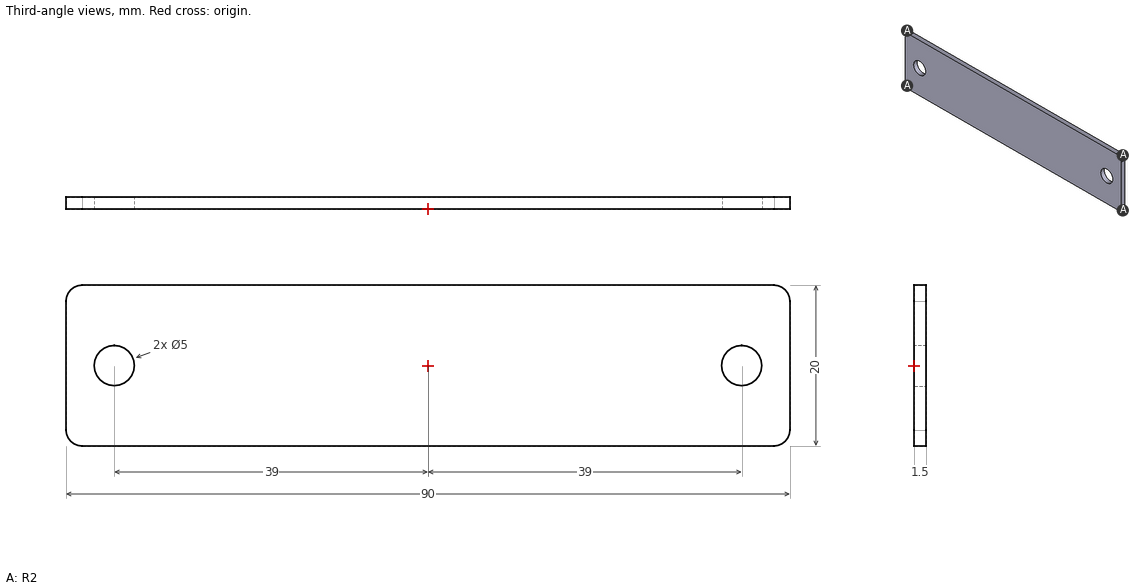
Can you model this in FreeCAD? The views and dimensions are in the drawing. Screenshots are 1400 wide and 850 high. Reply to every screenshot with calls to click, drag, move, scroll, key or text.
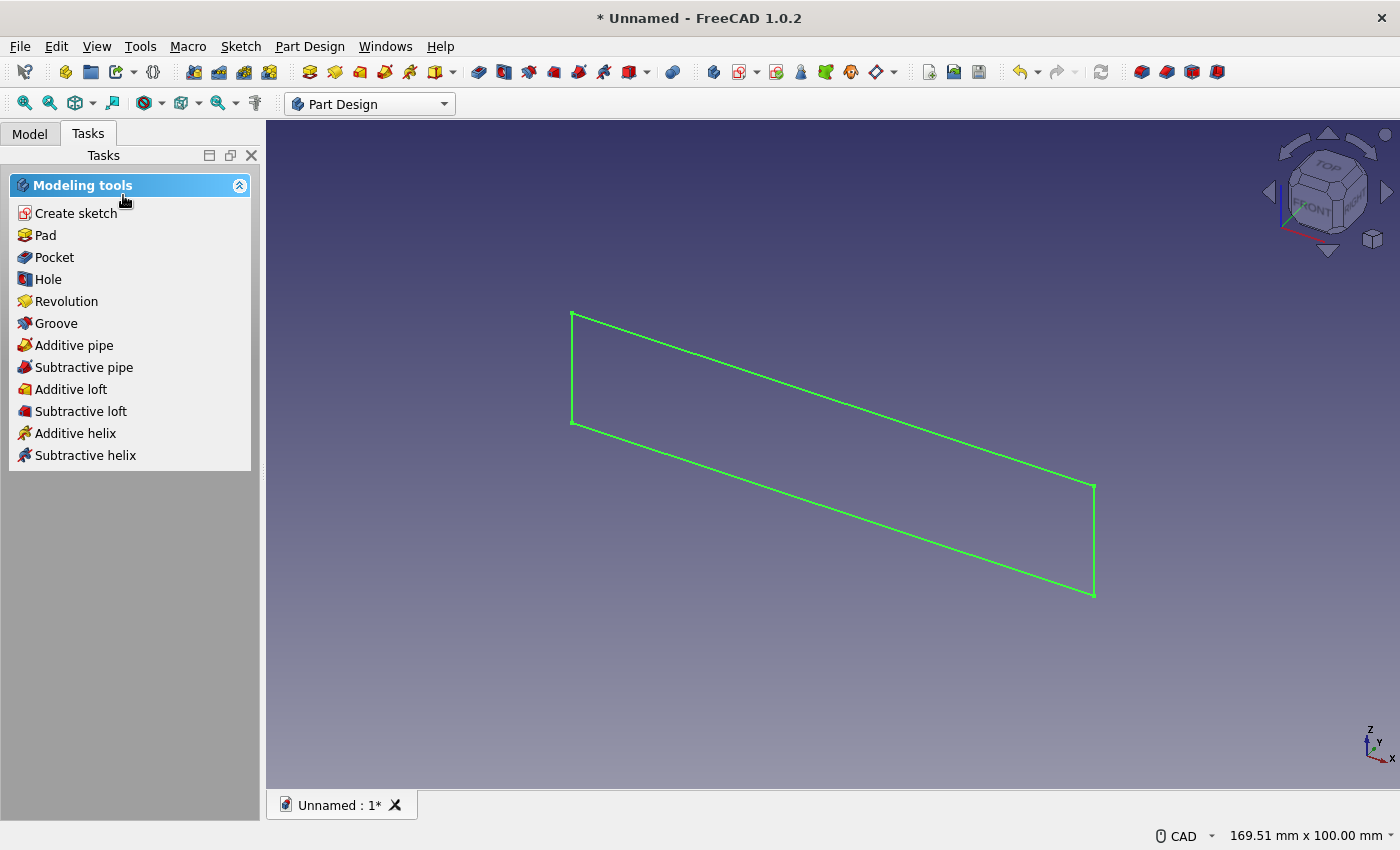
click(310, 72)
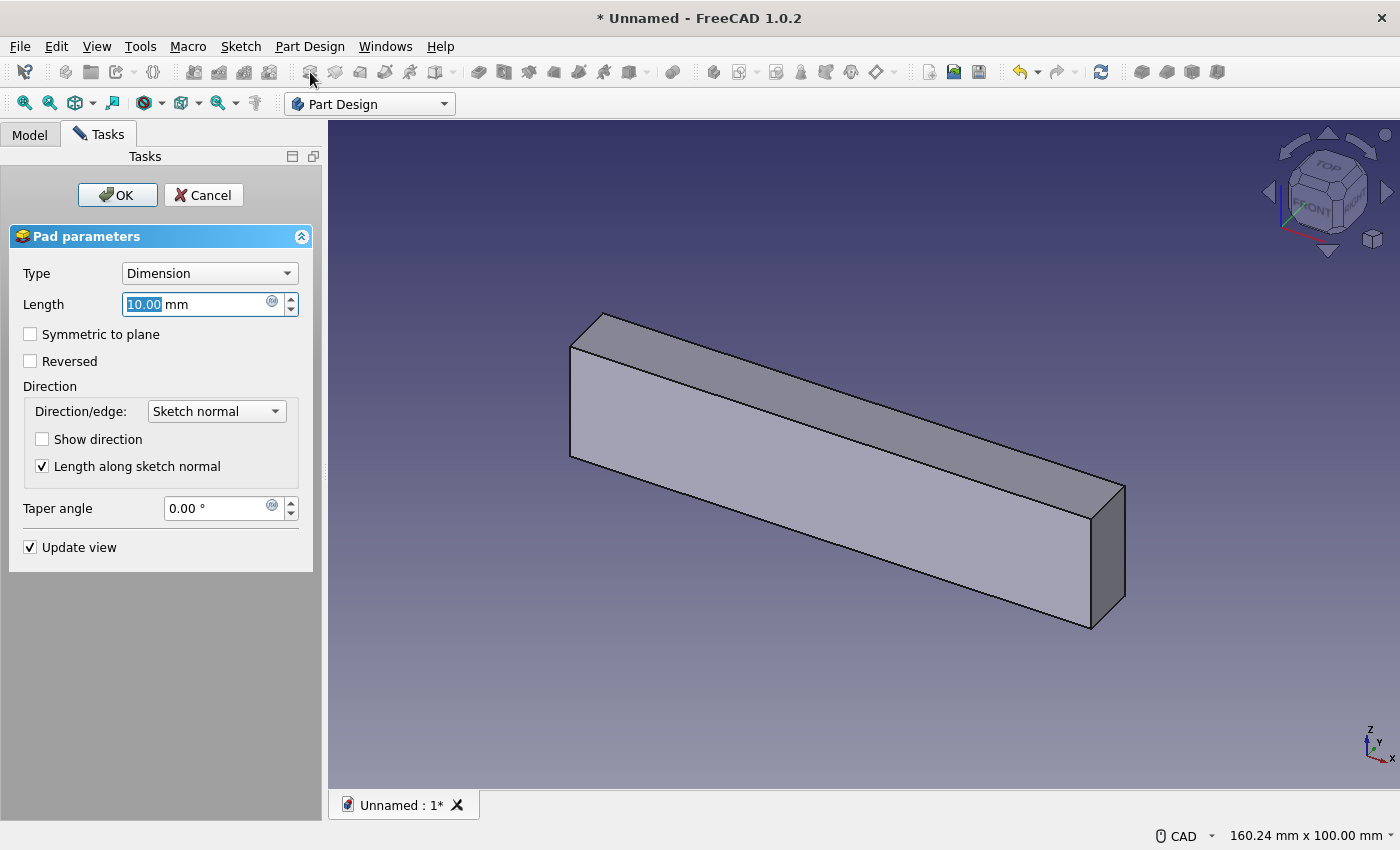
text(1.5)
key(Tab)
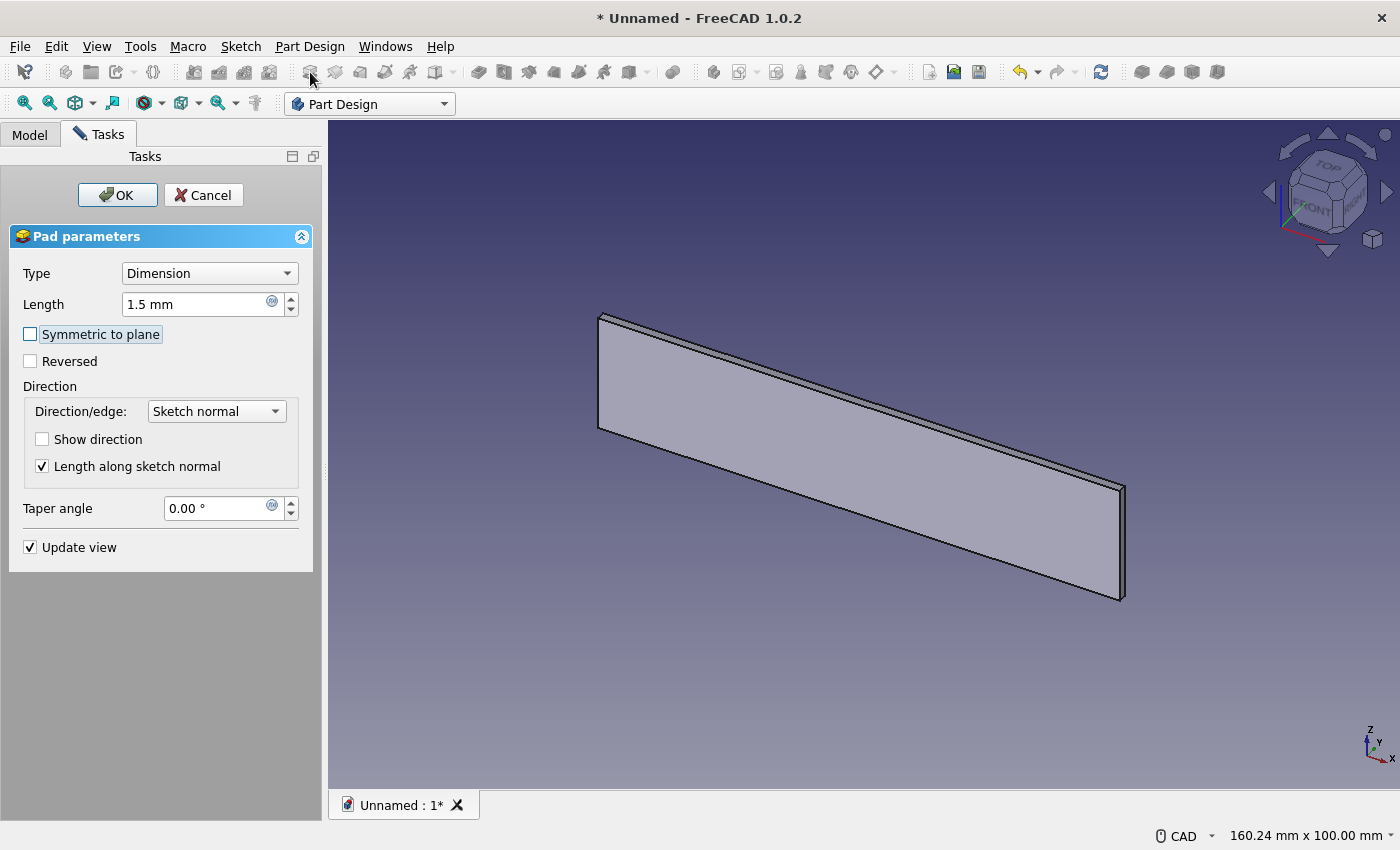
click(31, 361)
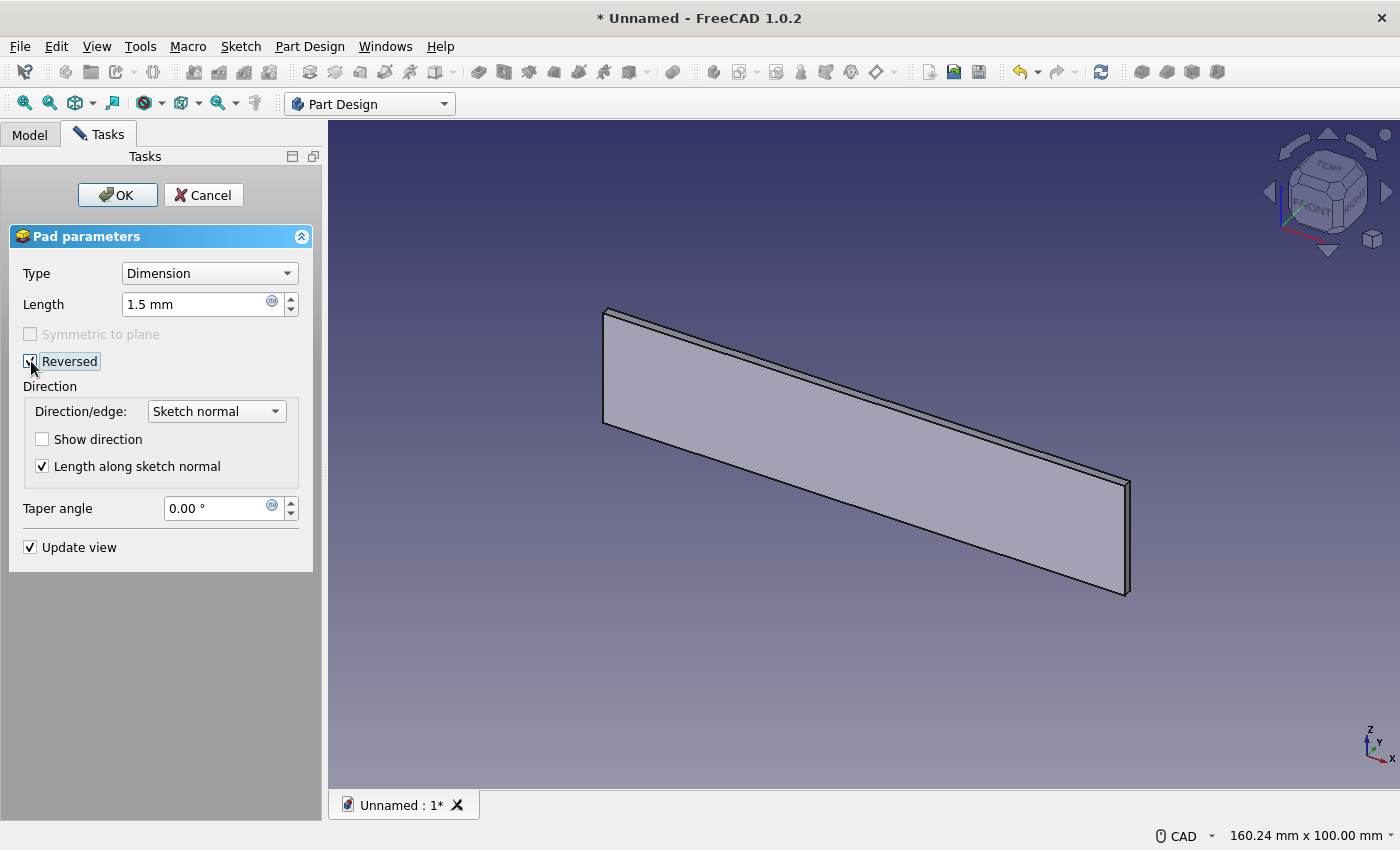
click(118, 195)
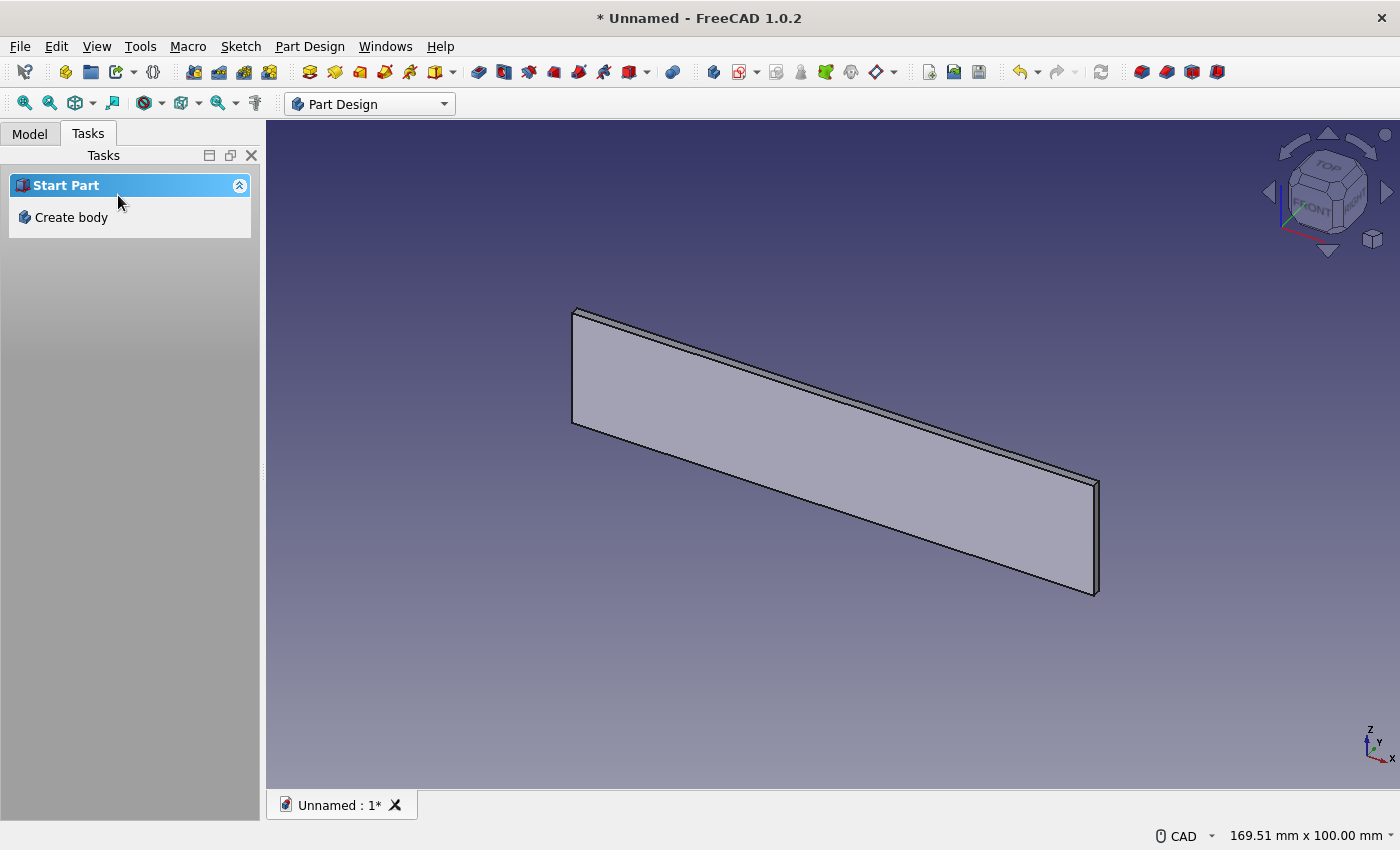
key(4)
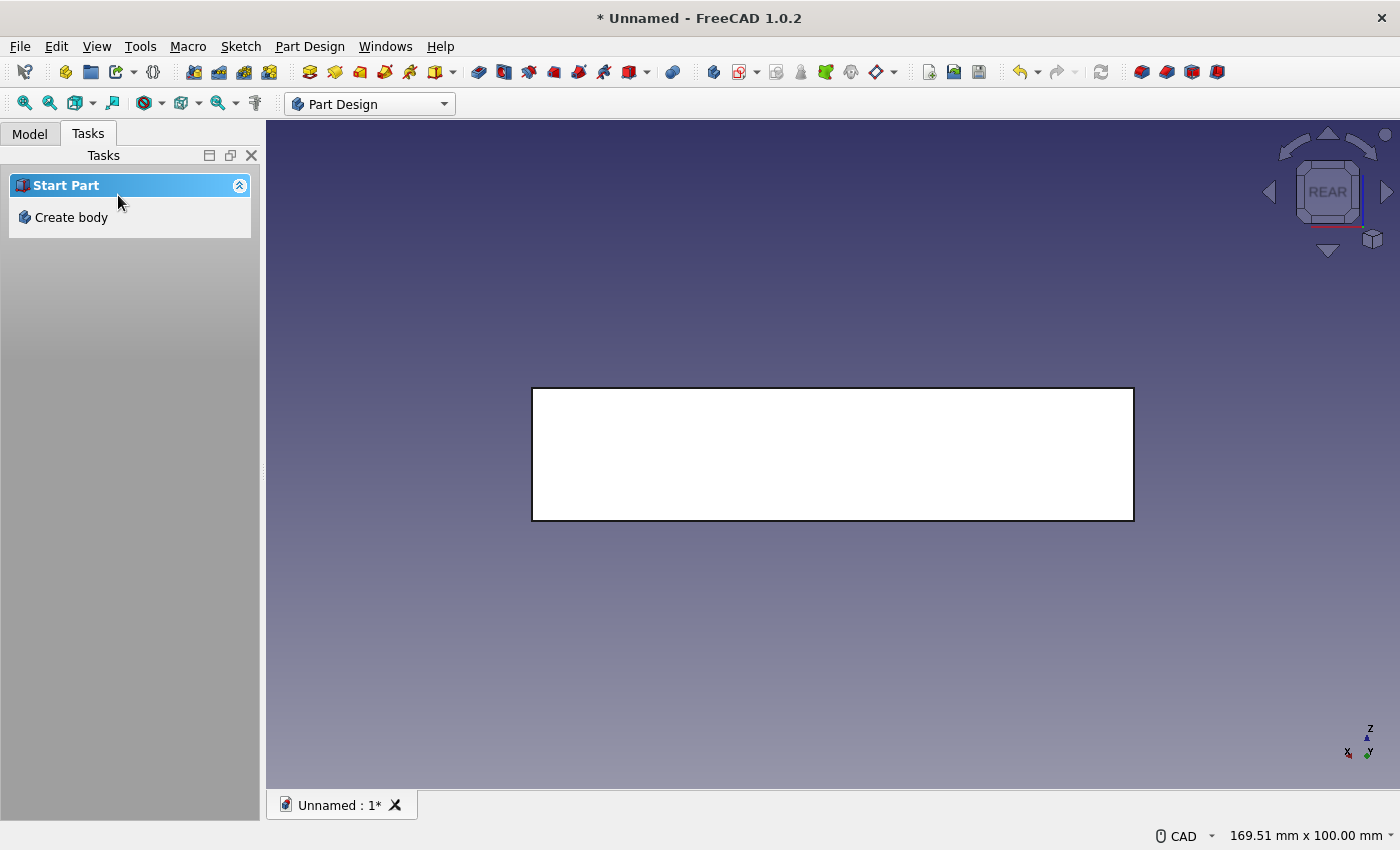
click(661, 453)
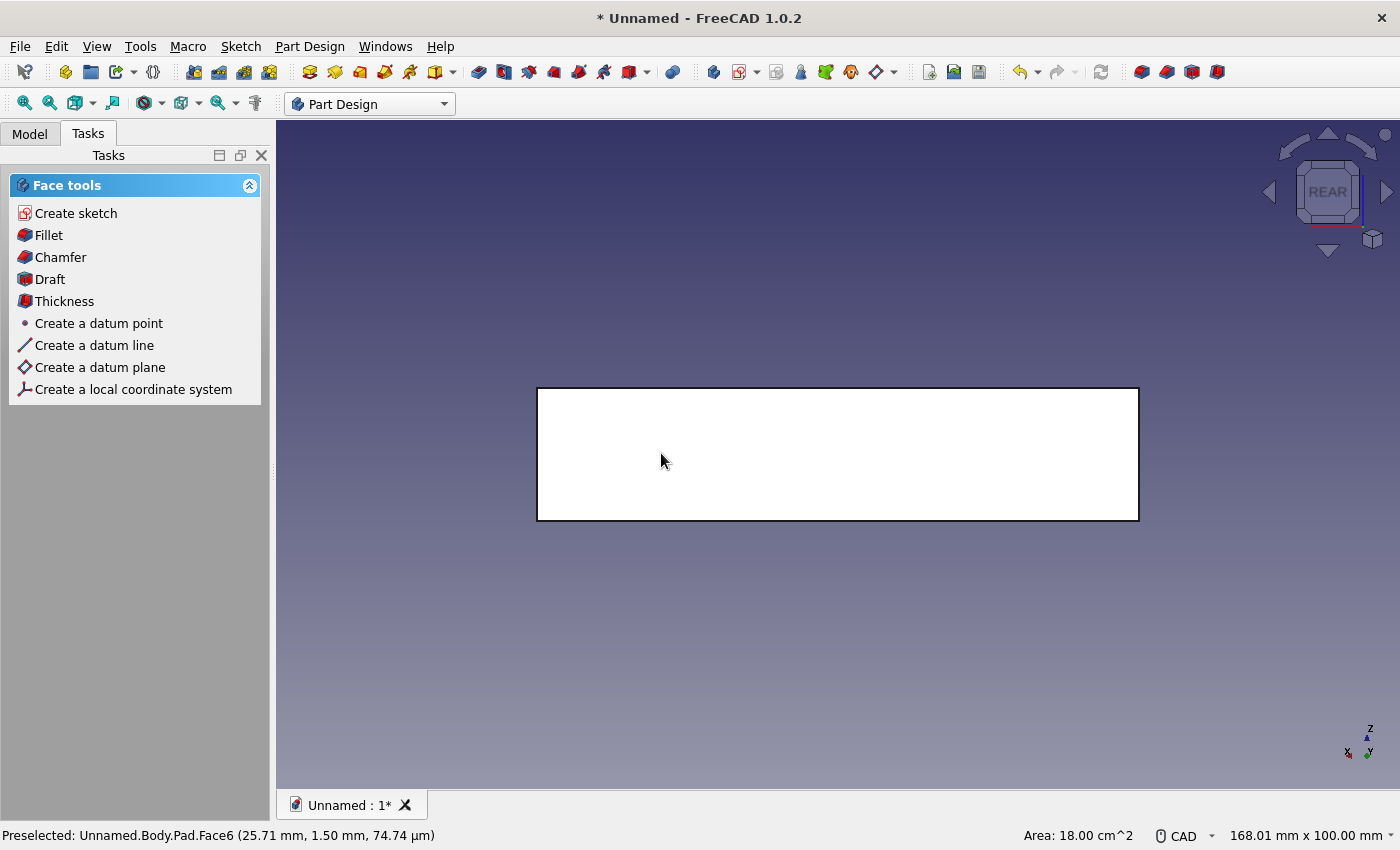
click(738, 72)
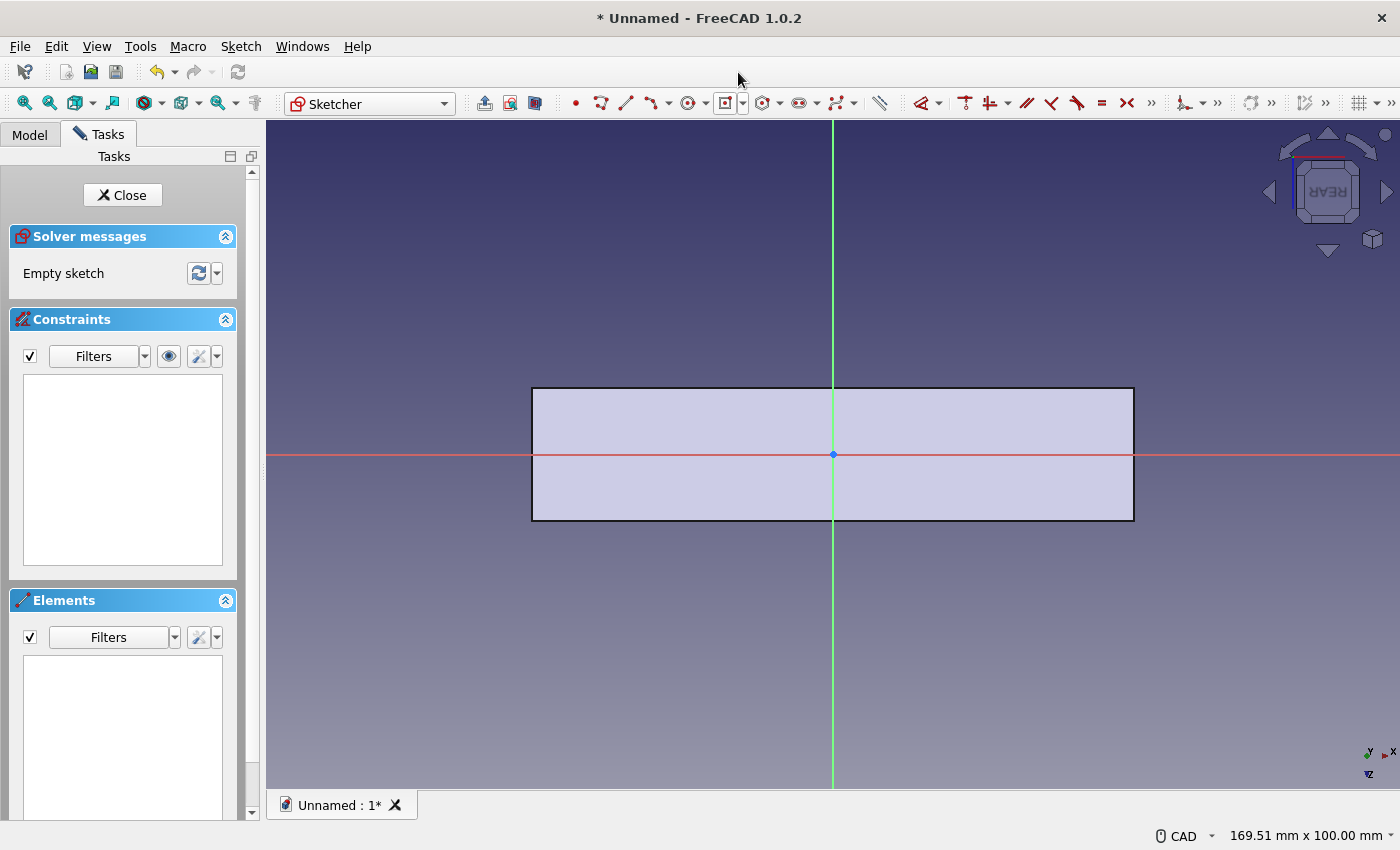
click(688, 104)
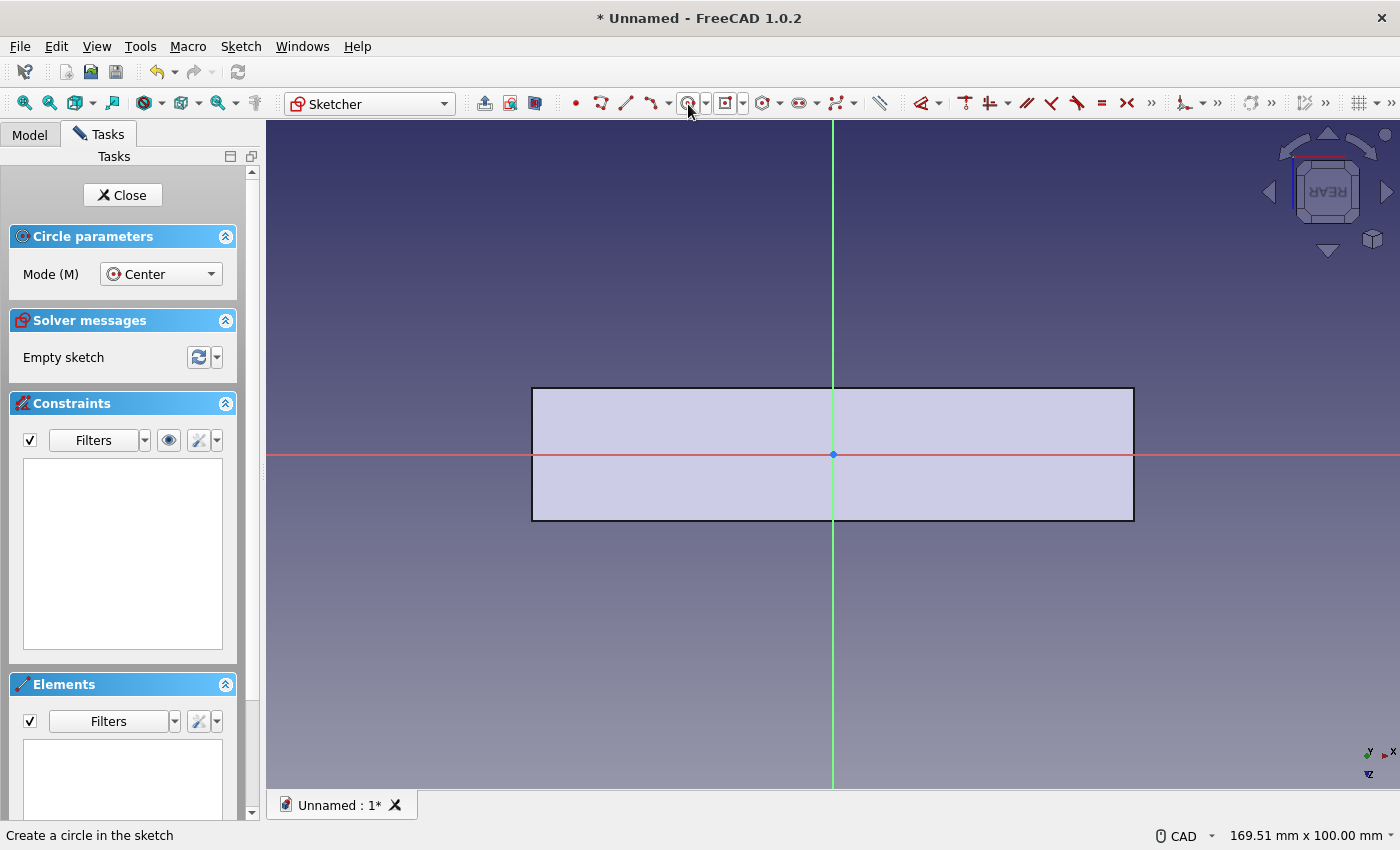
scroll(572, 455, up, 2)